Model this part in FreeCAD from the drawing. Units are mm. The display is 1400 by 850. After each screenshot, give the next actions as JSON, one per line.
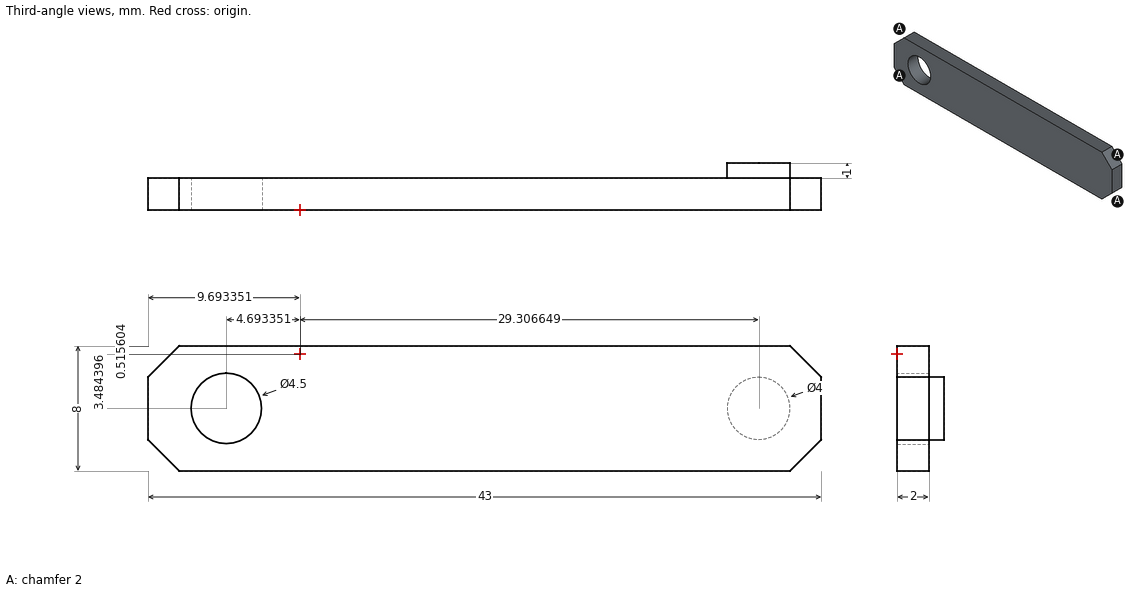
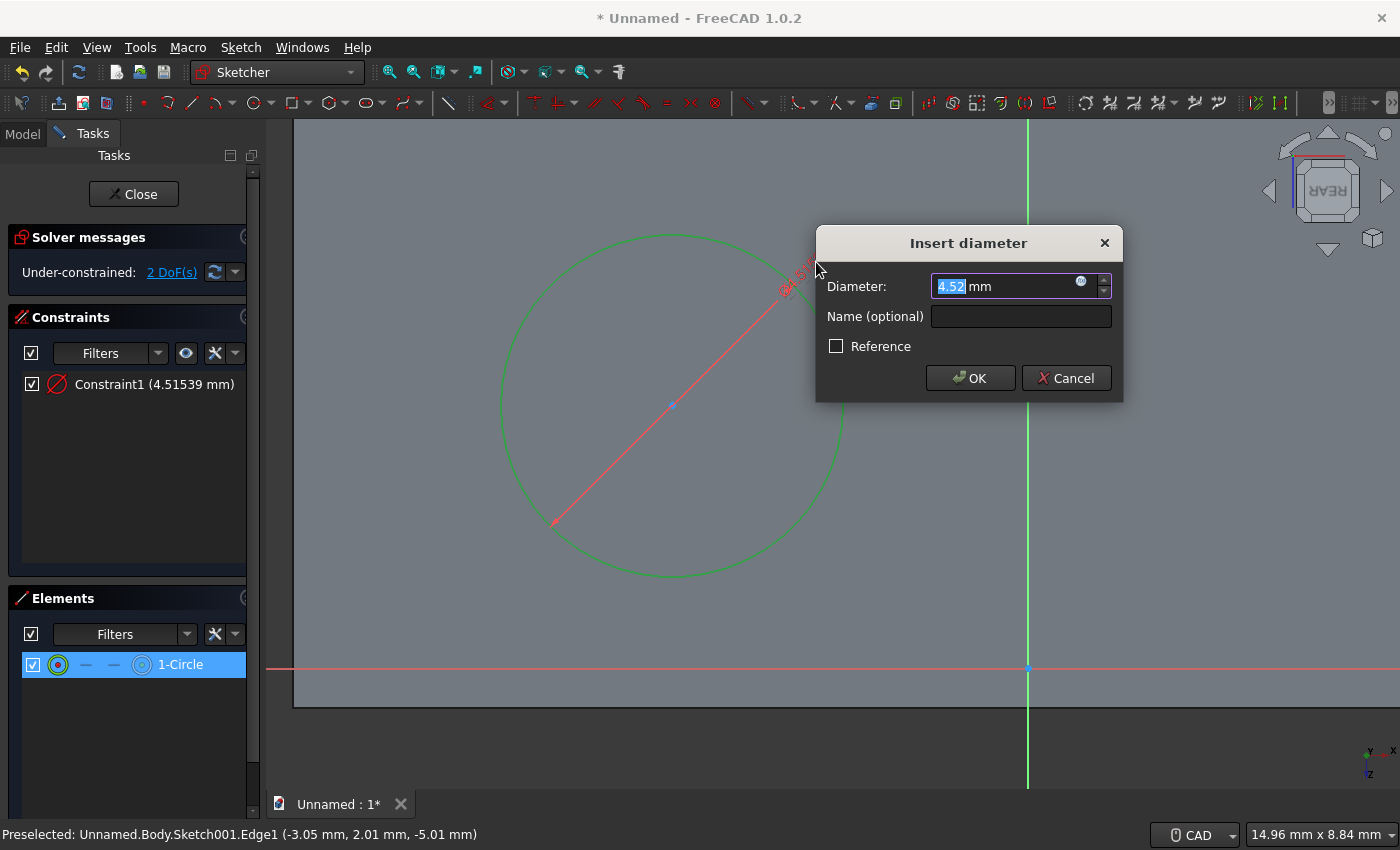
{"action": "type", "text": "4.5"}
{"action": "key", "text": "Return"}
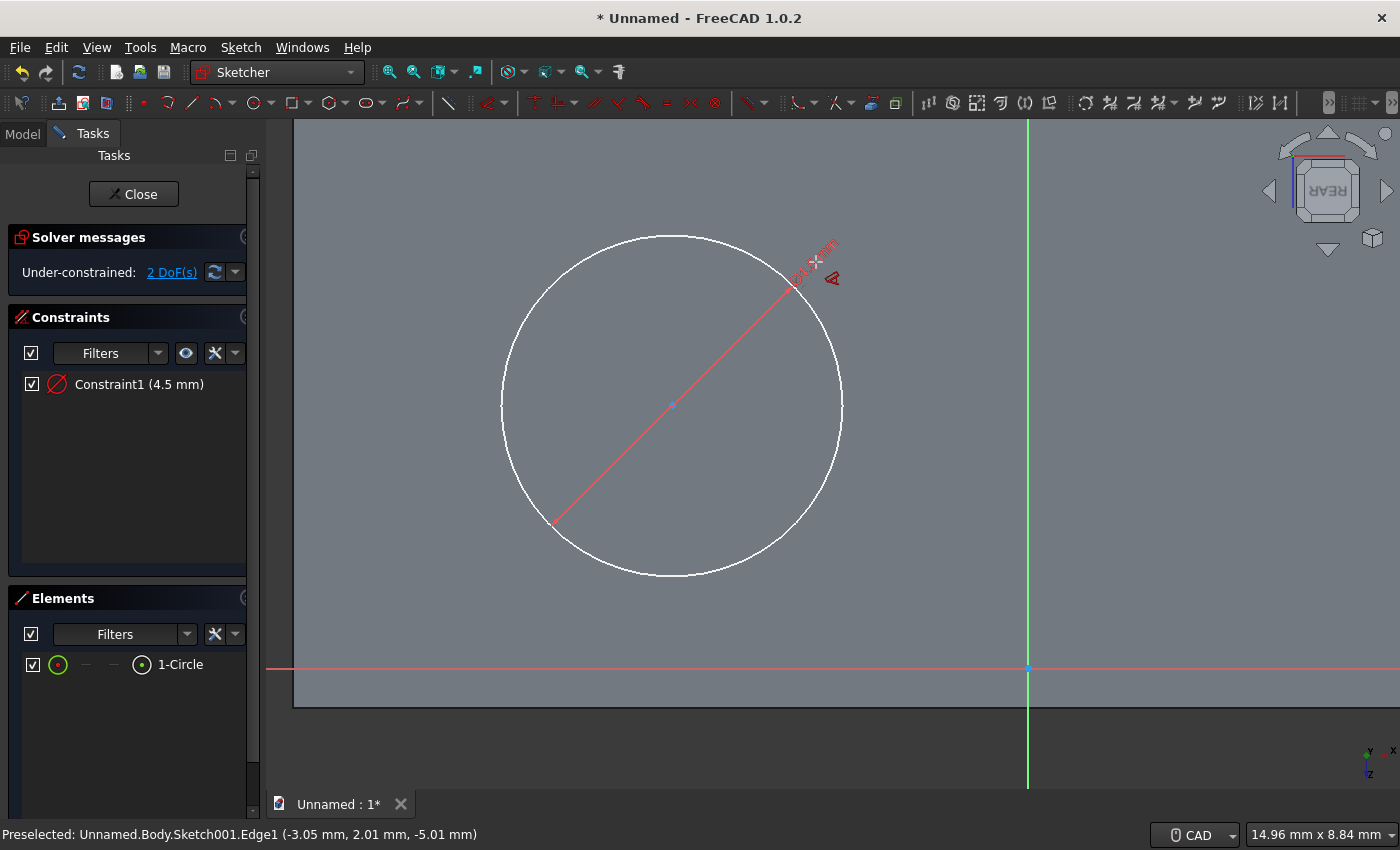
{"action": "left_click", "coordinate": [672, 406]}
{"action": "left_click", "coordinate": [850, 703]}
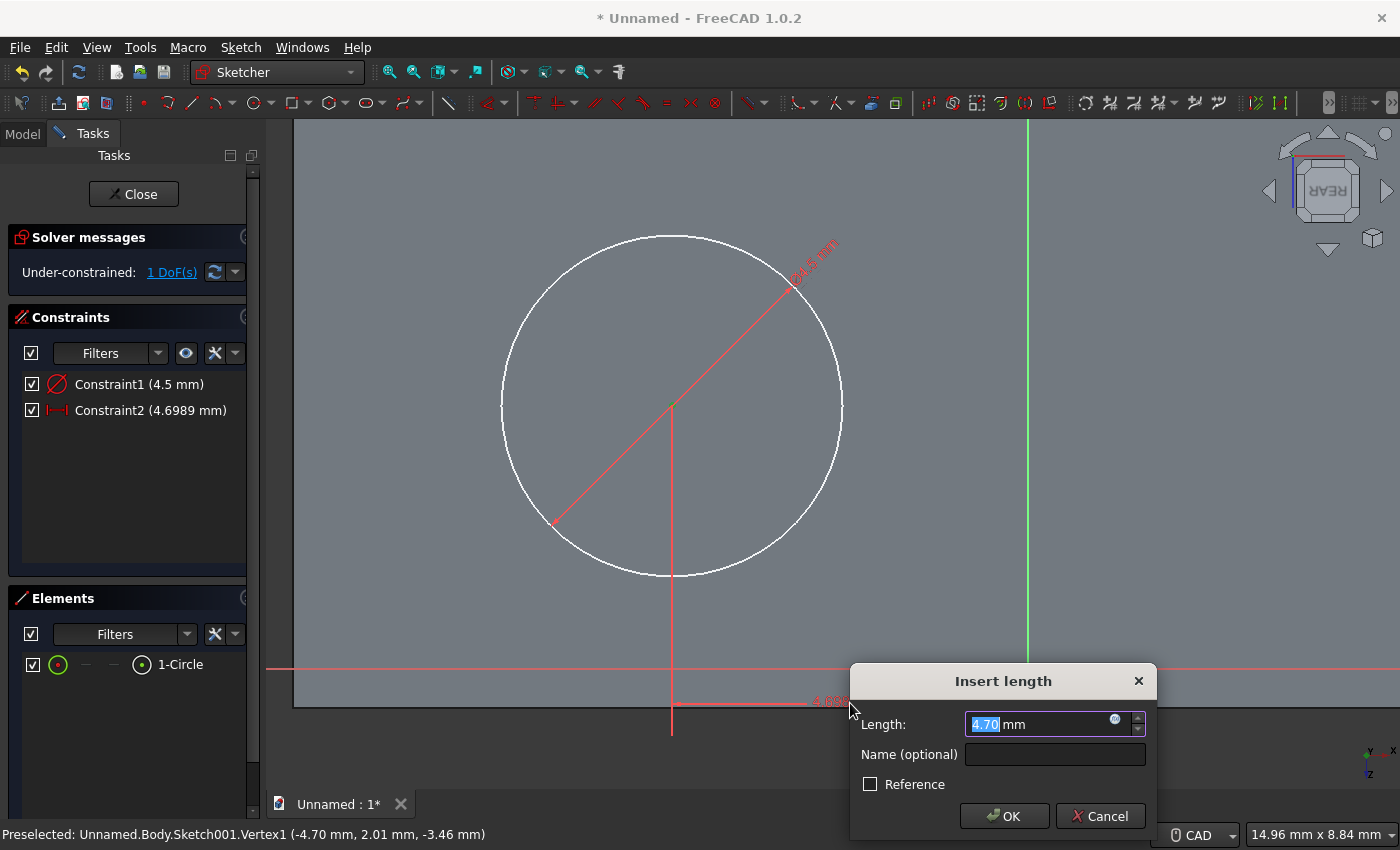
{"action": "type", "text": "4.693351"}
{"action": "key", "text": "Return"}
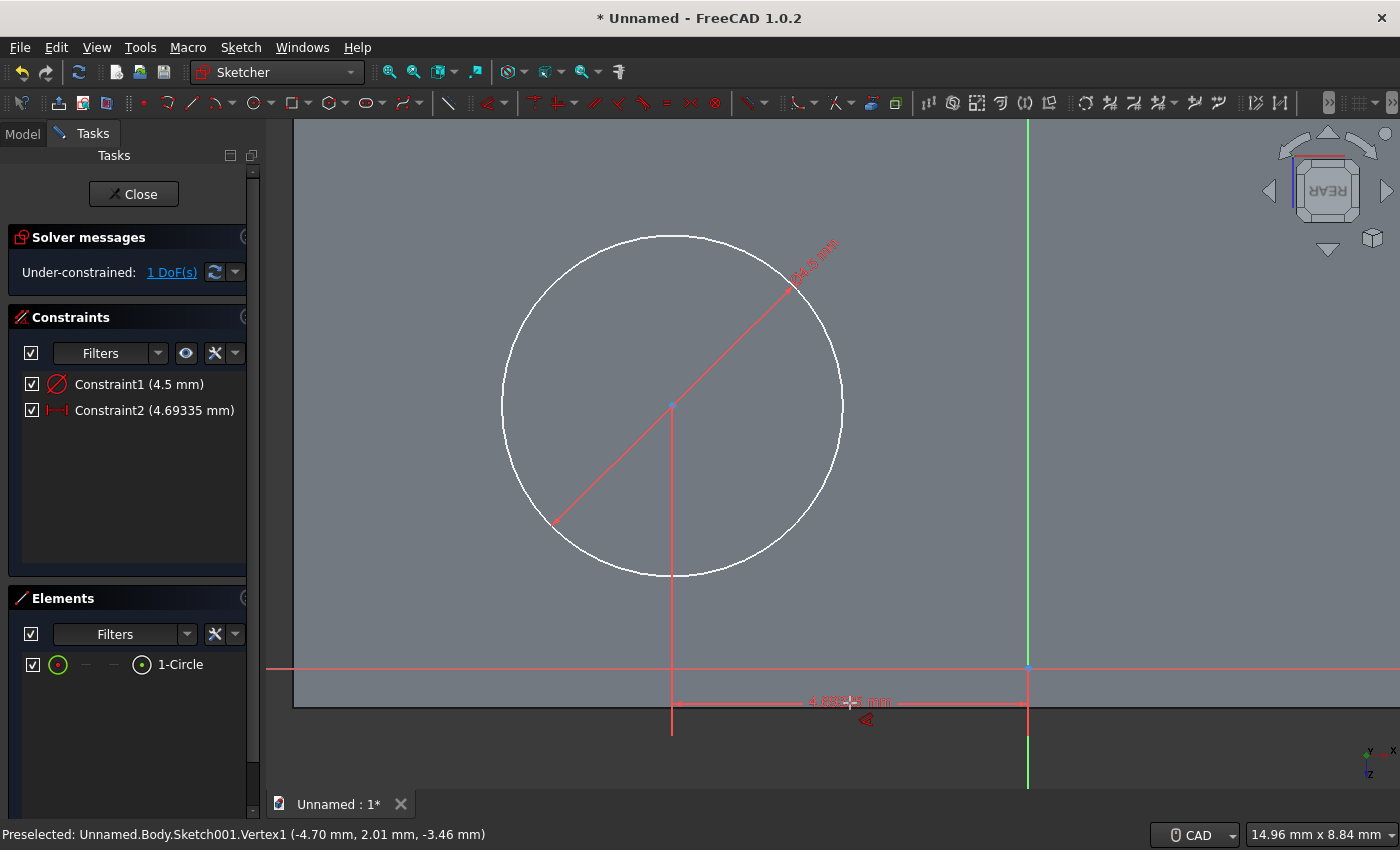
{"action": "left_click", "coordinate": [672, 406]}
{"action": "left_click", "coordinate": [1062, 537]}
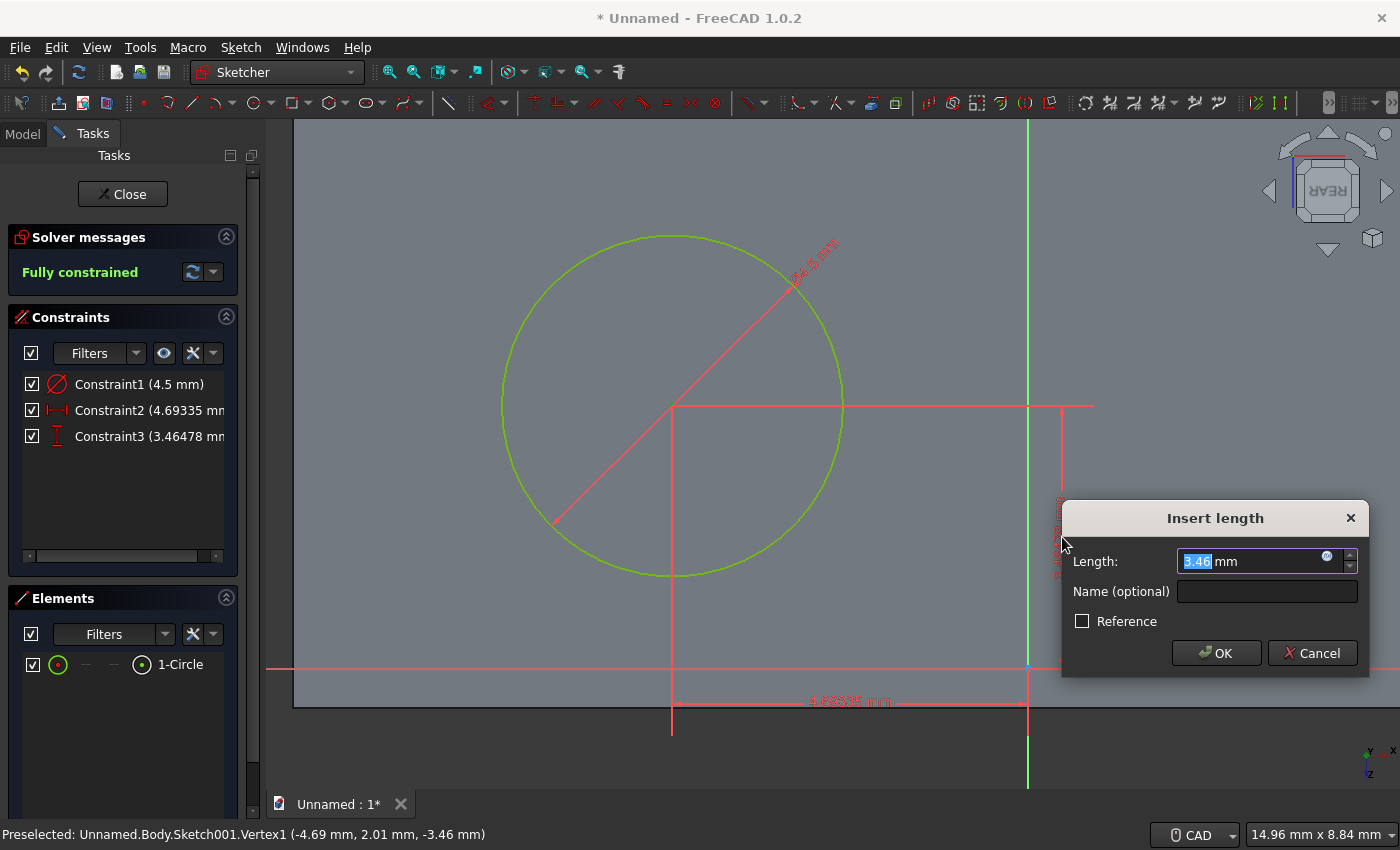
{"action": "type", "text": "3.484396"}
{"action": "key", "text": "Return"}
{"action": "key", "text": "Escape"}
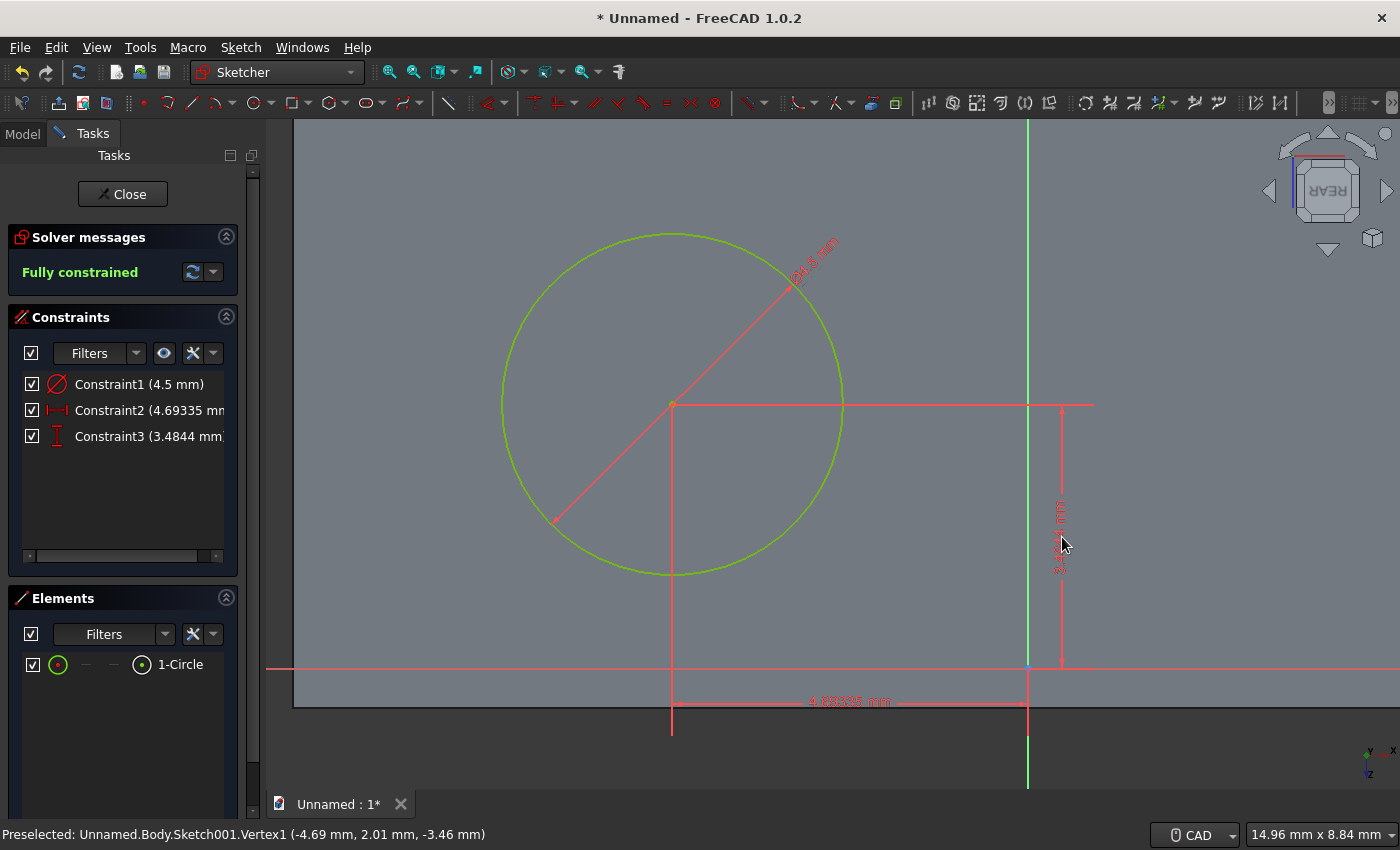
{"action": "left_click", "coordinate": [123, 194]}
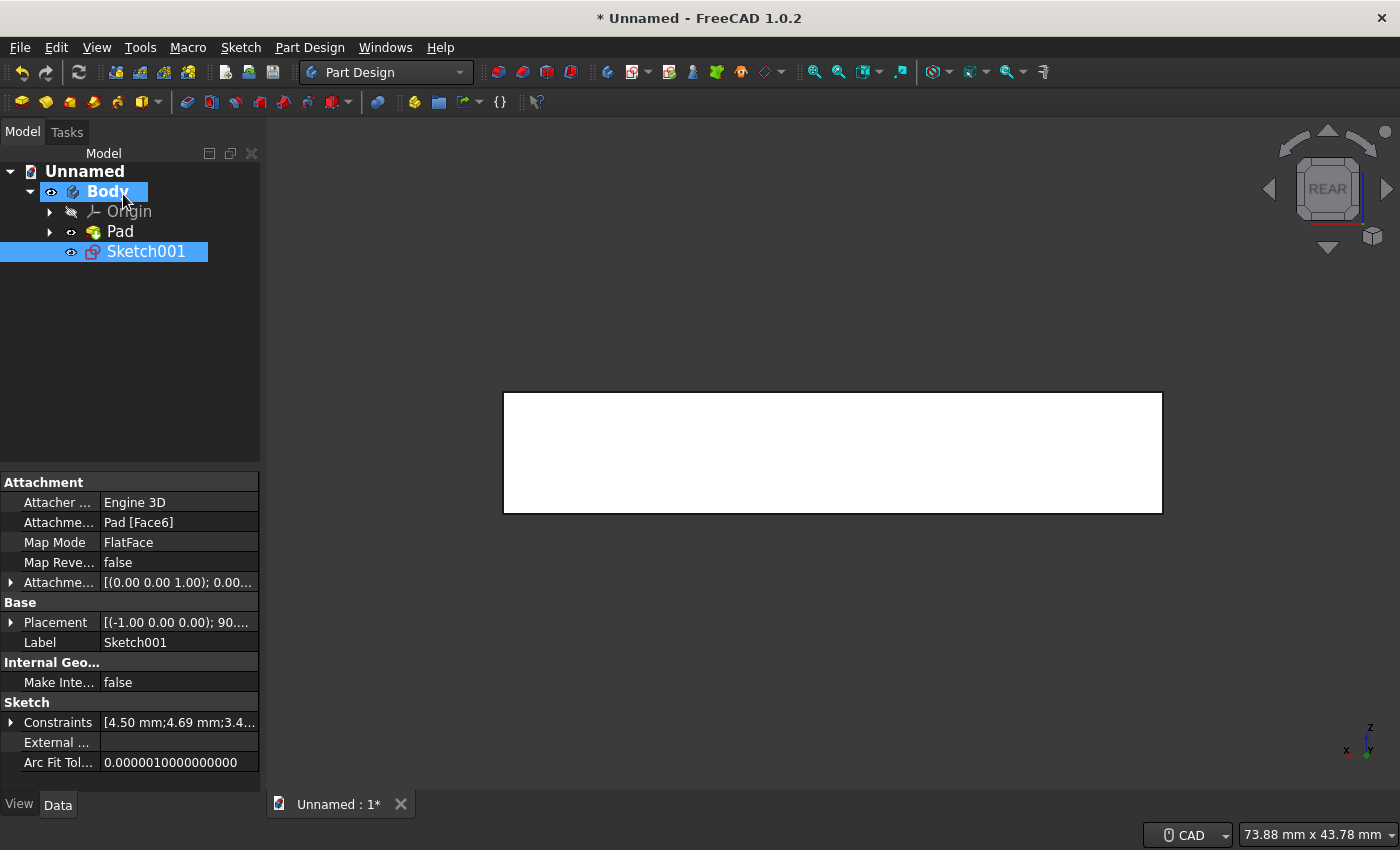
{"action": "left_click", "coordinate": [188, 102]}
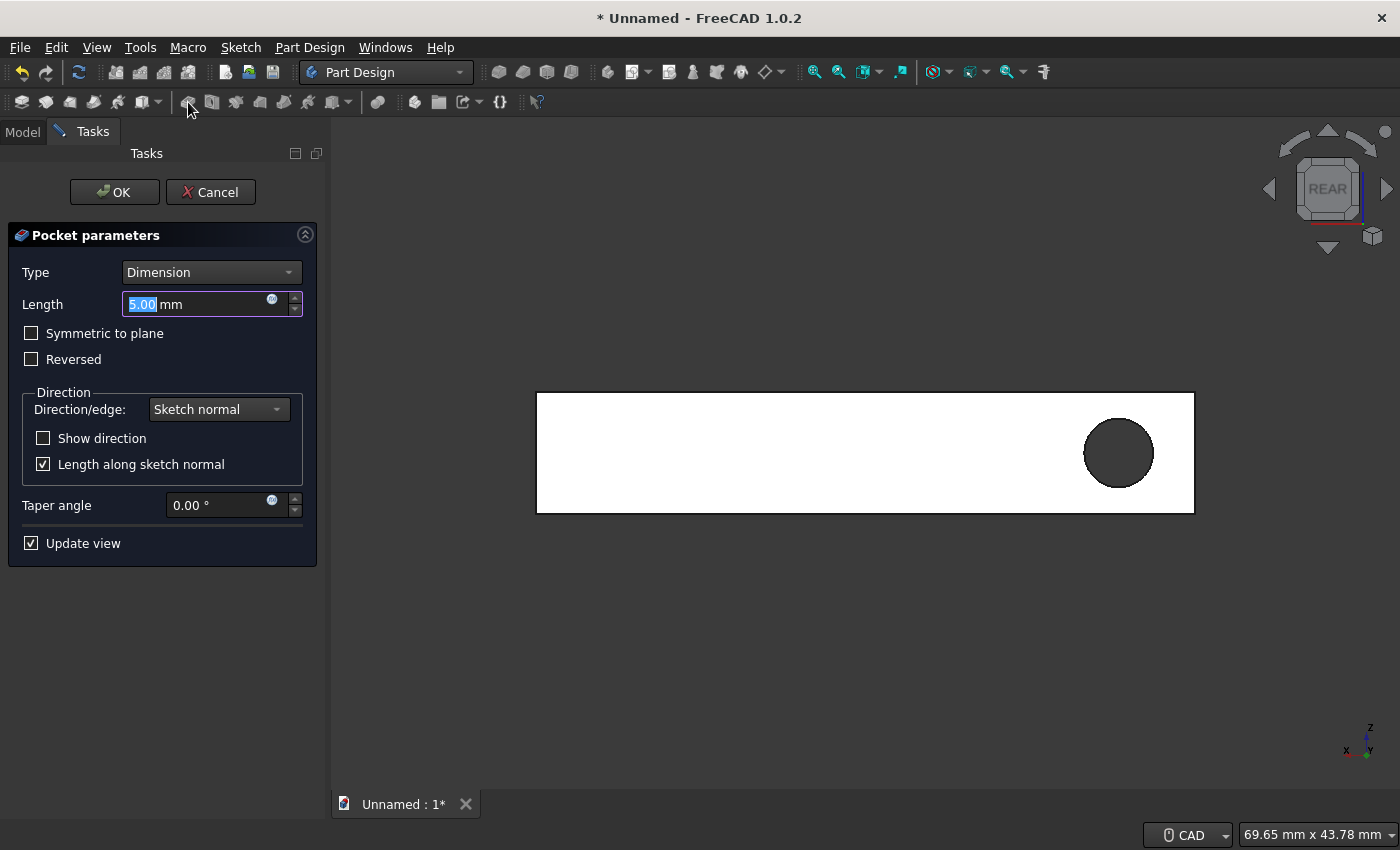
{"action": "left_click", "coordinate": [212, 272]}